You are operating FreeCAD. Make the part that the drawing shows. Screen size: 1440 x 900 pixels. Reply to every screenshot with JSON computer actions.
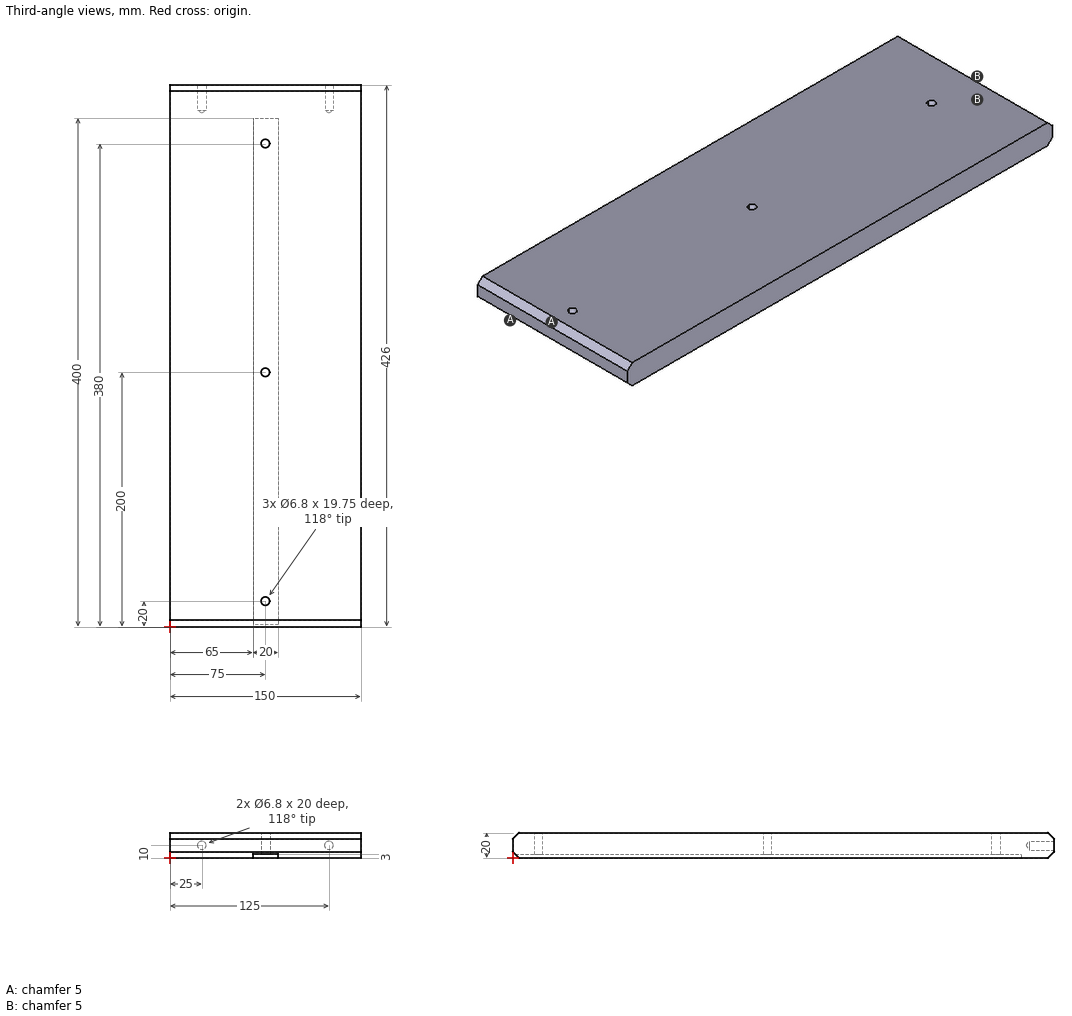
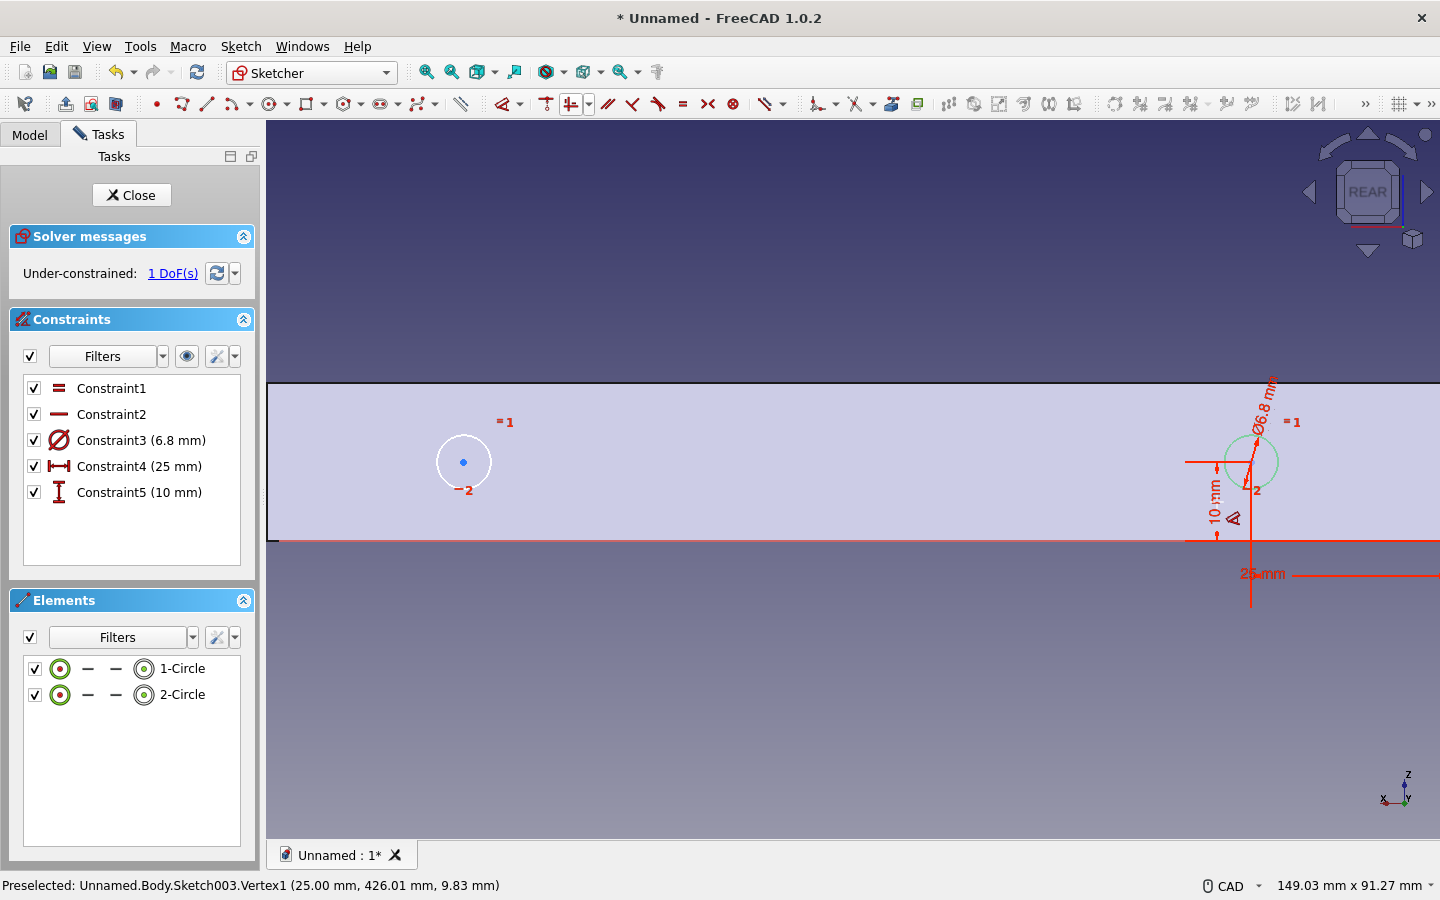
{"action": "left_click", "coordinate": [464, 462]}
{"action": "left_click", "coordinate": [869, 575]}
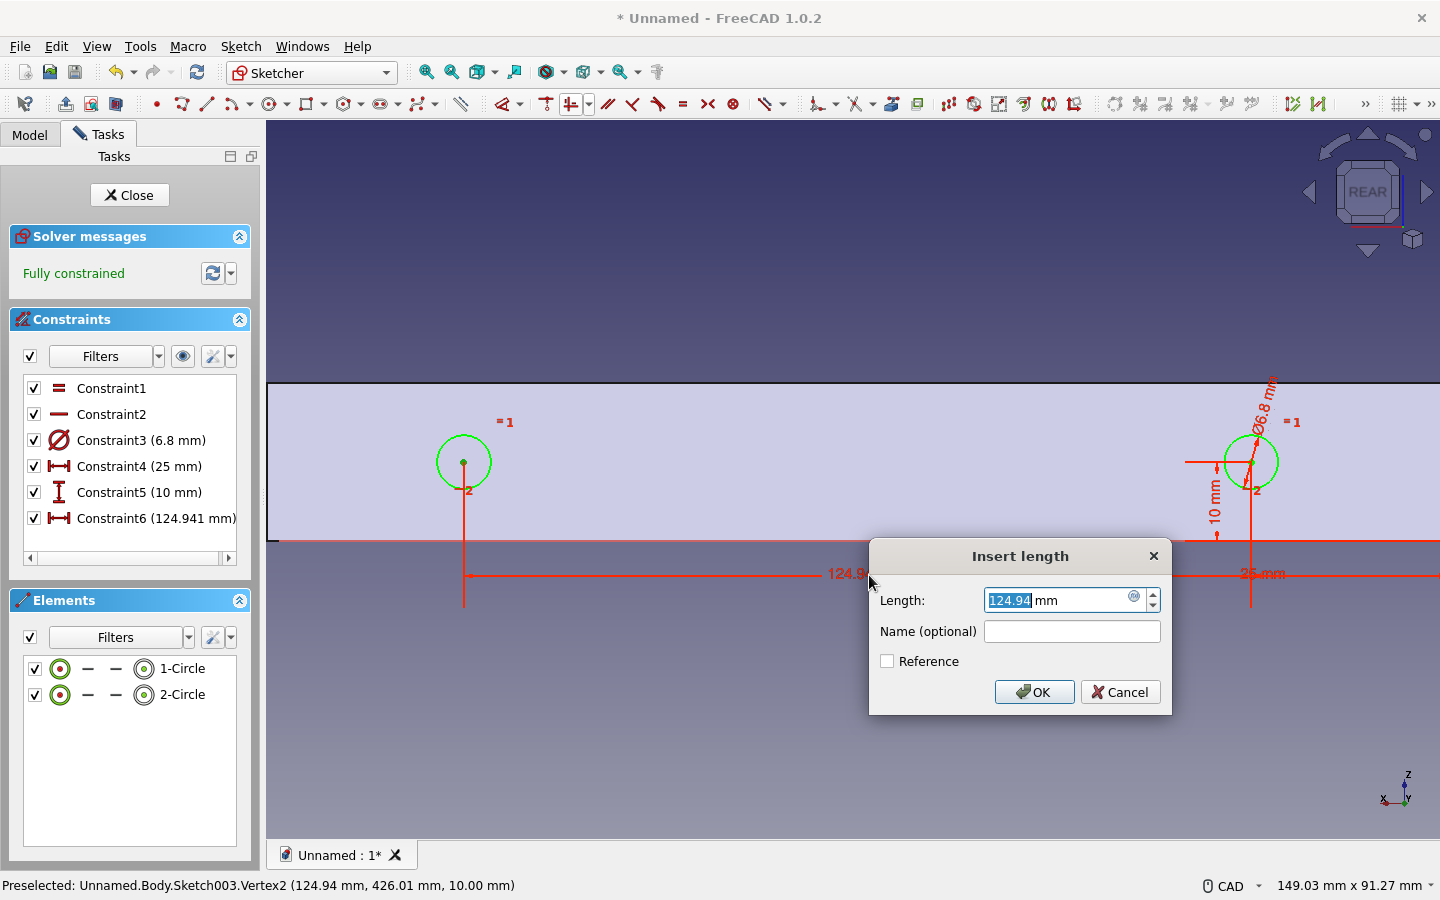
{"action": "type", "text": "125"}
{"action": "key", "text": "Return"}
{"action": "key", "text": "Escape"}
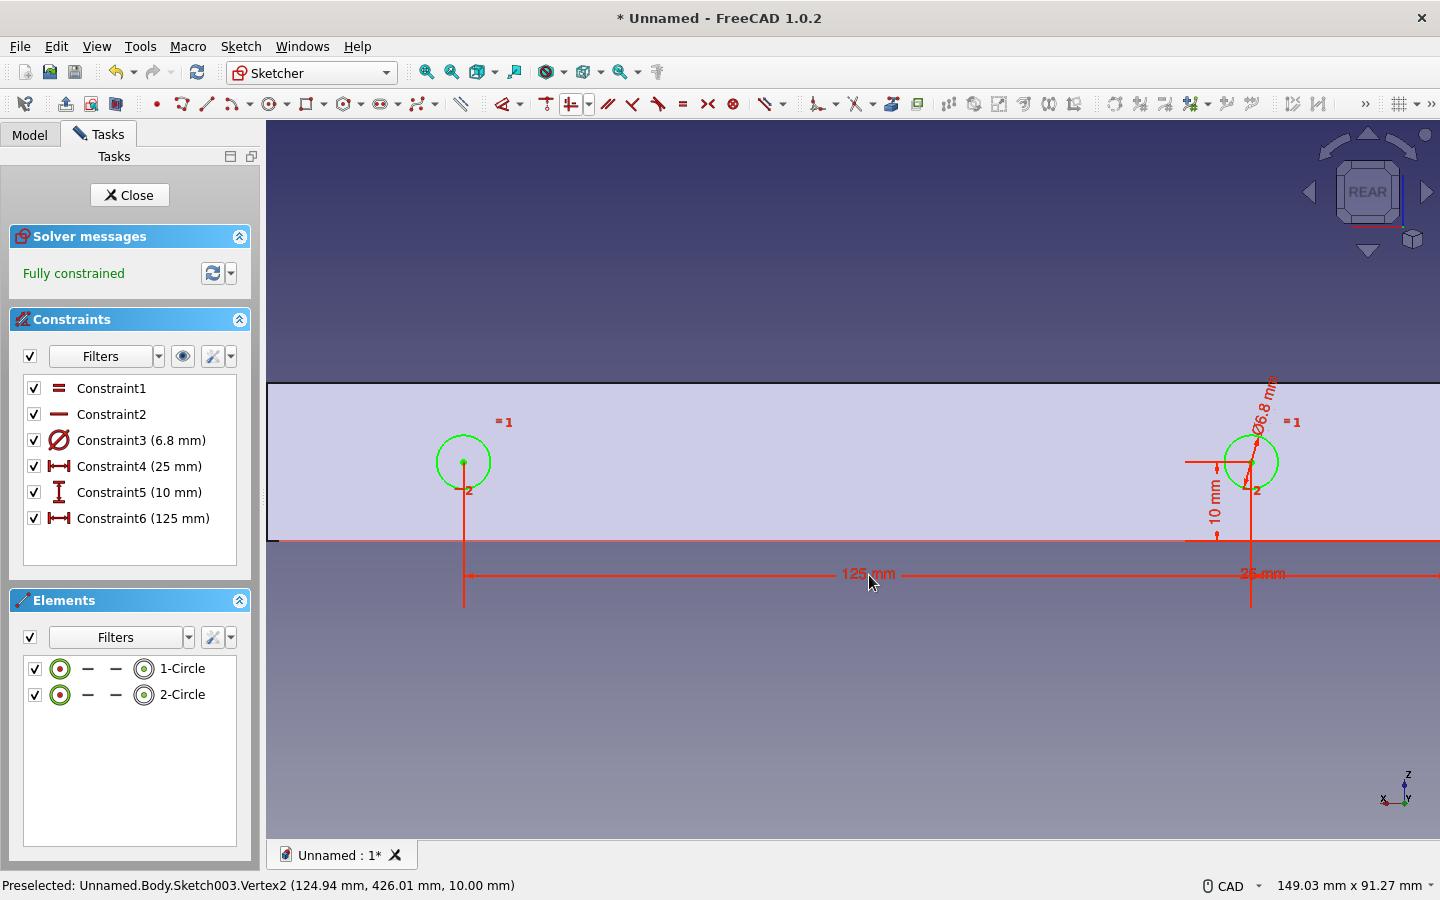
{"action": "left_click", "coordinate": [130, 195]}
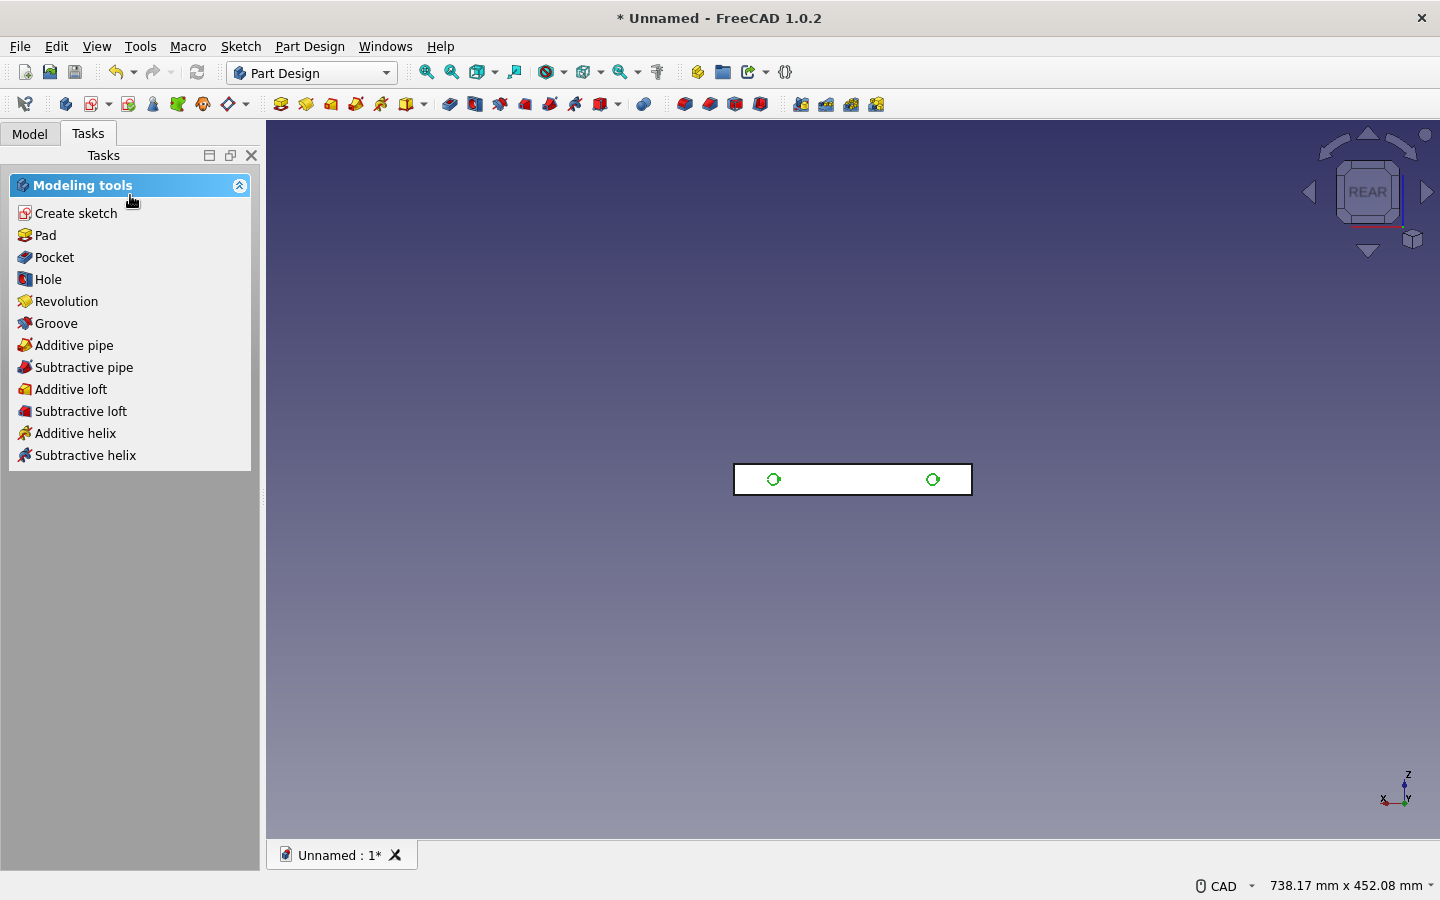
{"action": "left_click", "coordinate": [475, 104]}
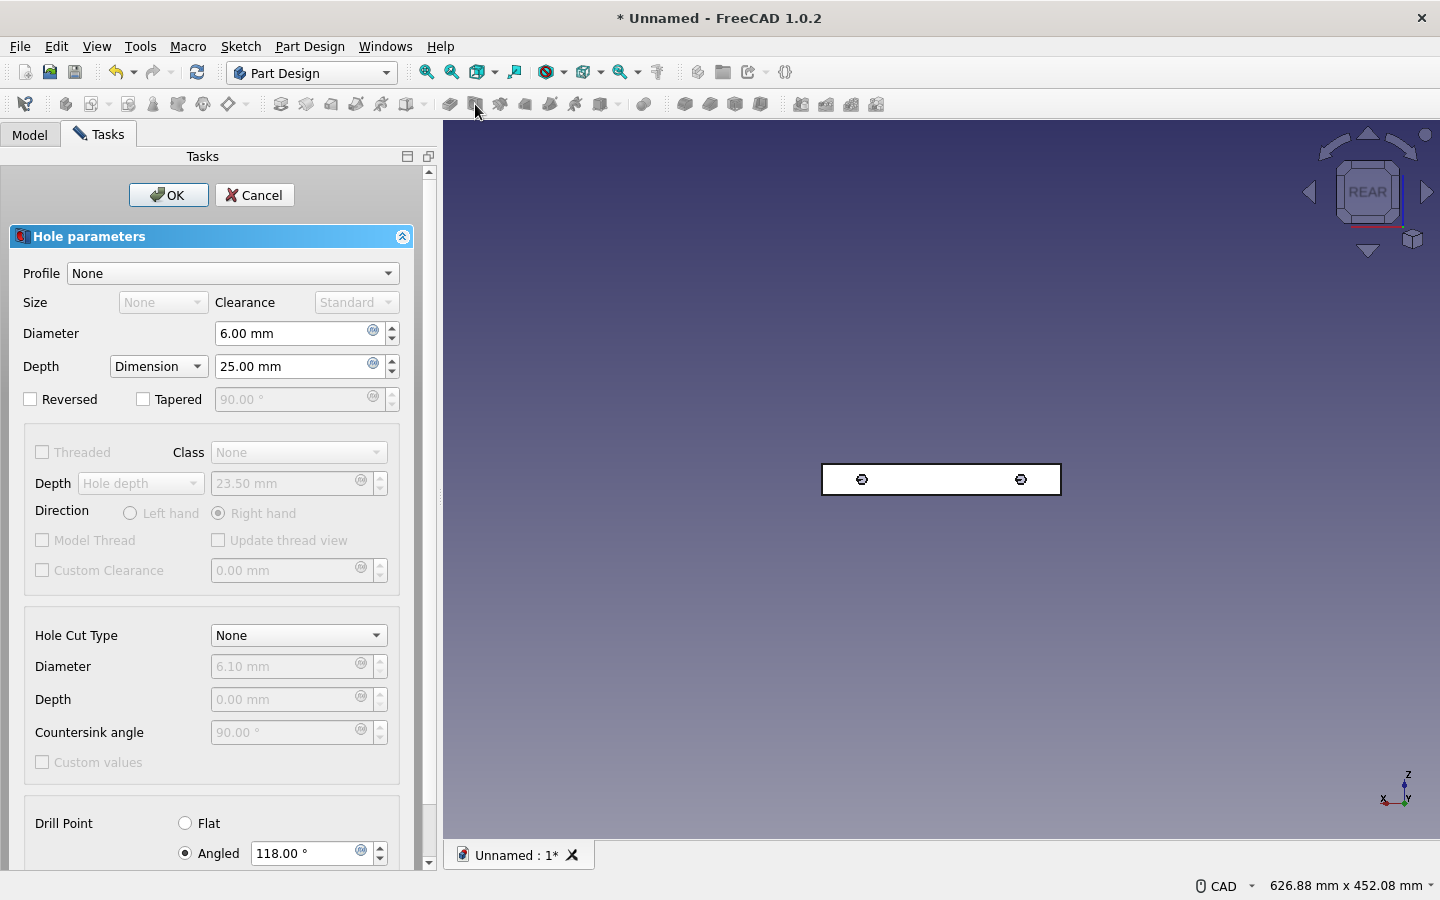
{"action": "triple_click", "coordinate": [300, 334]}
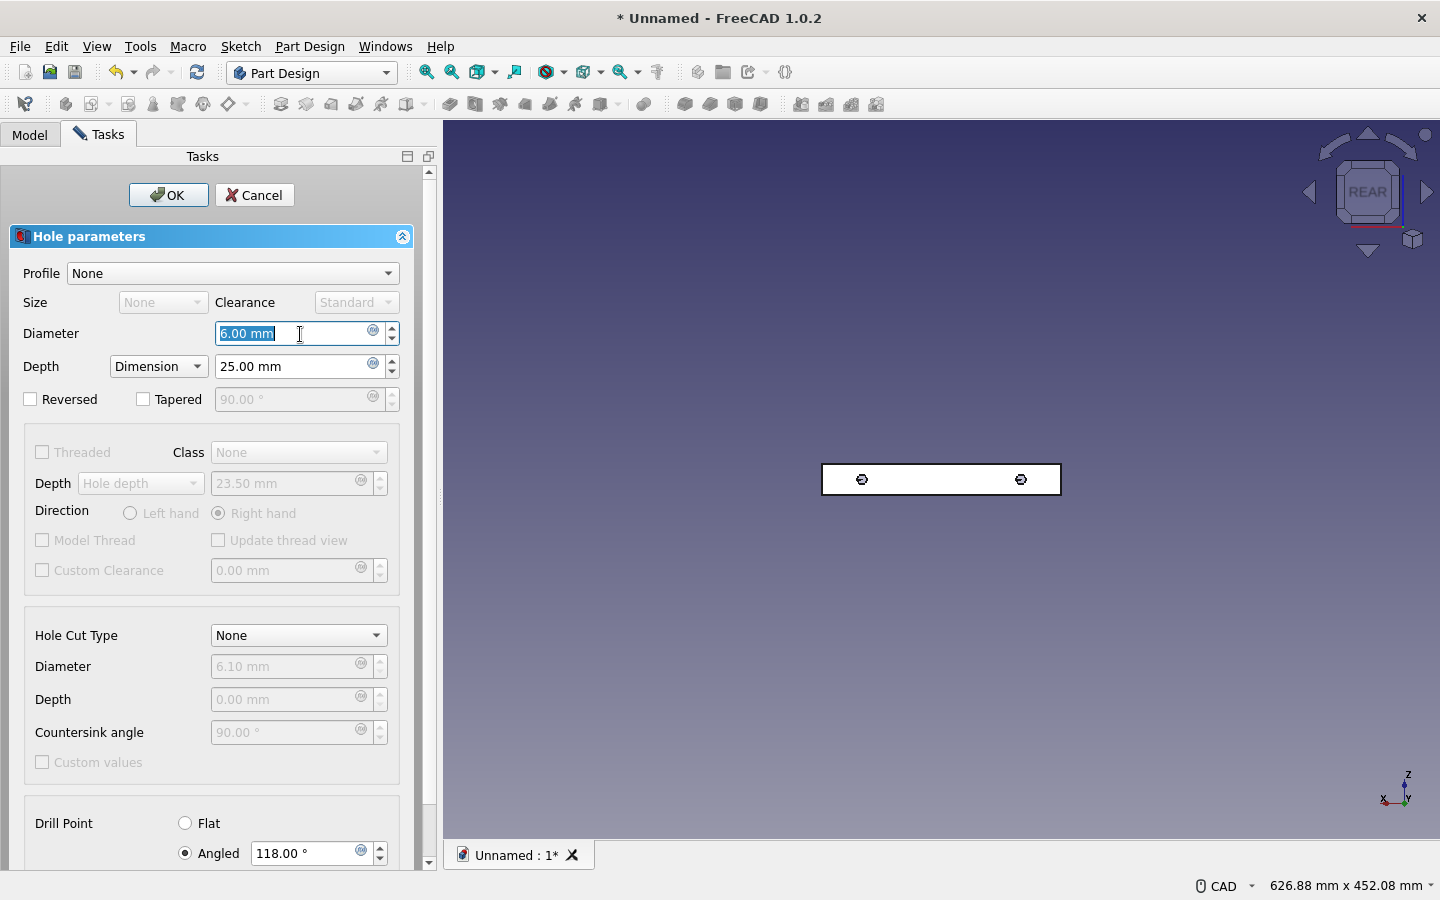
{"action": "type", "text": "6.8"}
{"action": "key", "text": "Tab"}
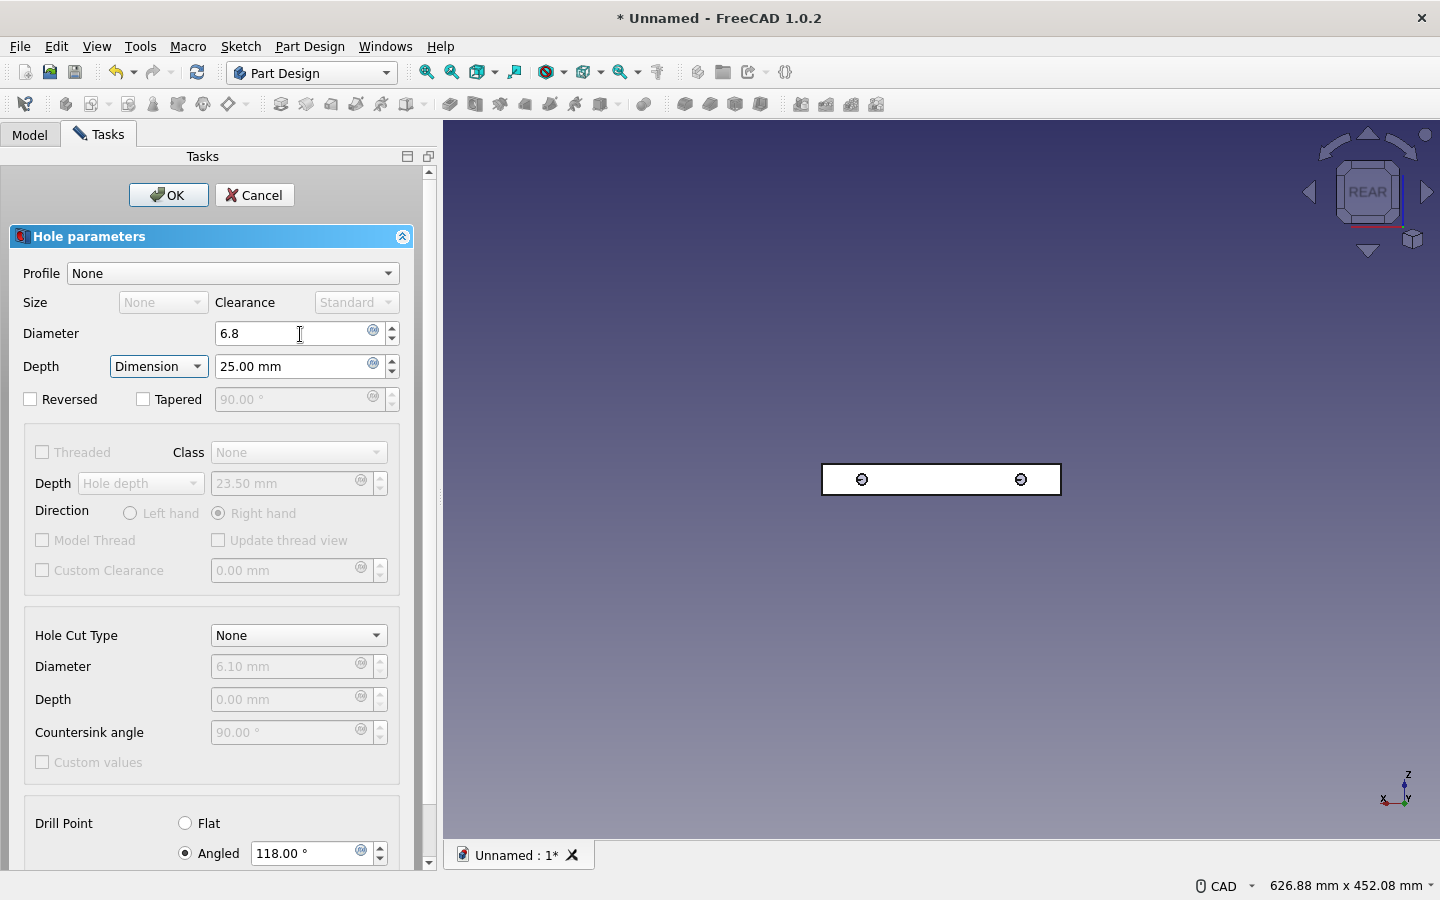
{"action": "triple_click", "coordinate": [300, 366]}